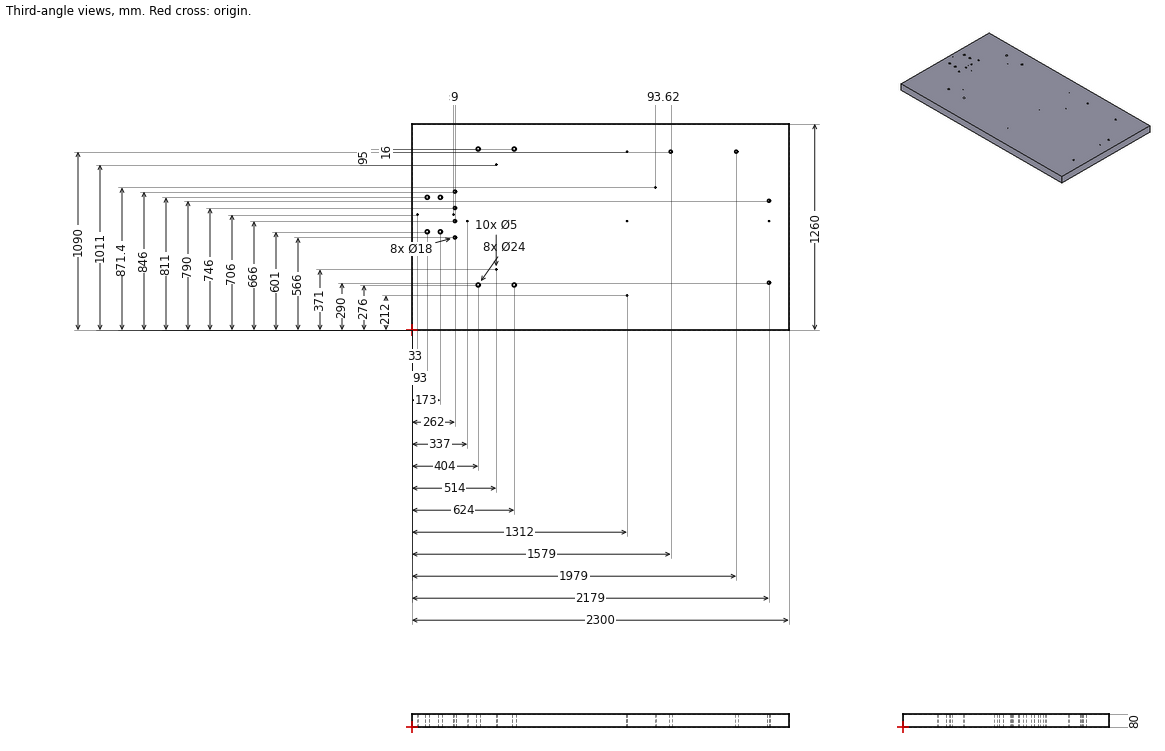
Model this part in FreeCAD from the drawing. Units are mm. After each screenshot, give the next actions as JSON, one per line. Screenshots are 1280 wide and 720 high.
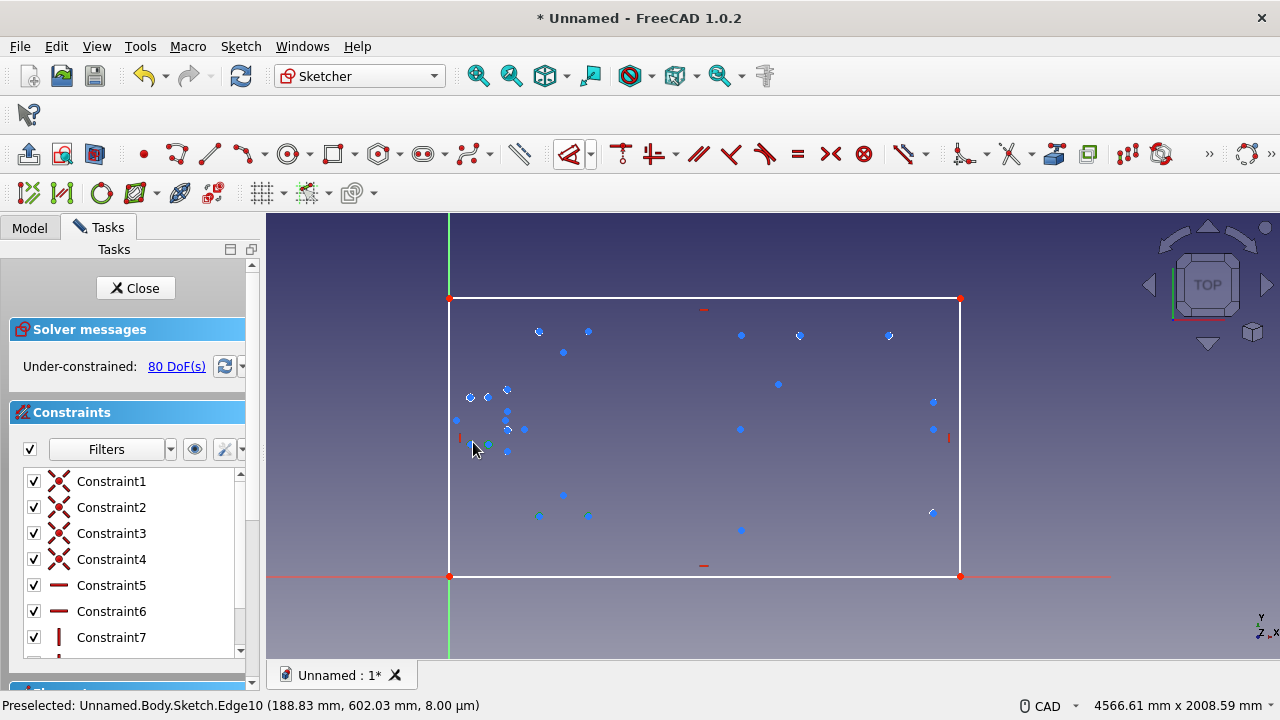
{"action": "scroll", "coordinate": [473, 395], "scroll_direction": "up", "scroll_amount": 8}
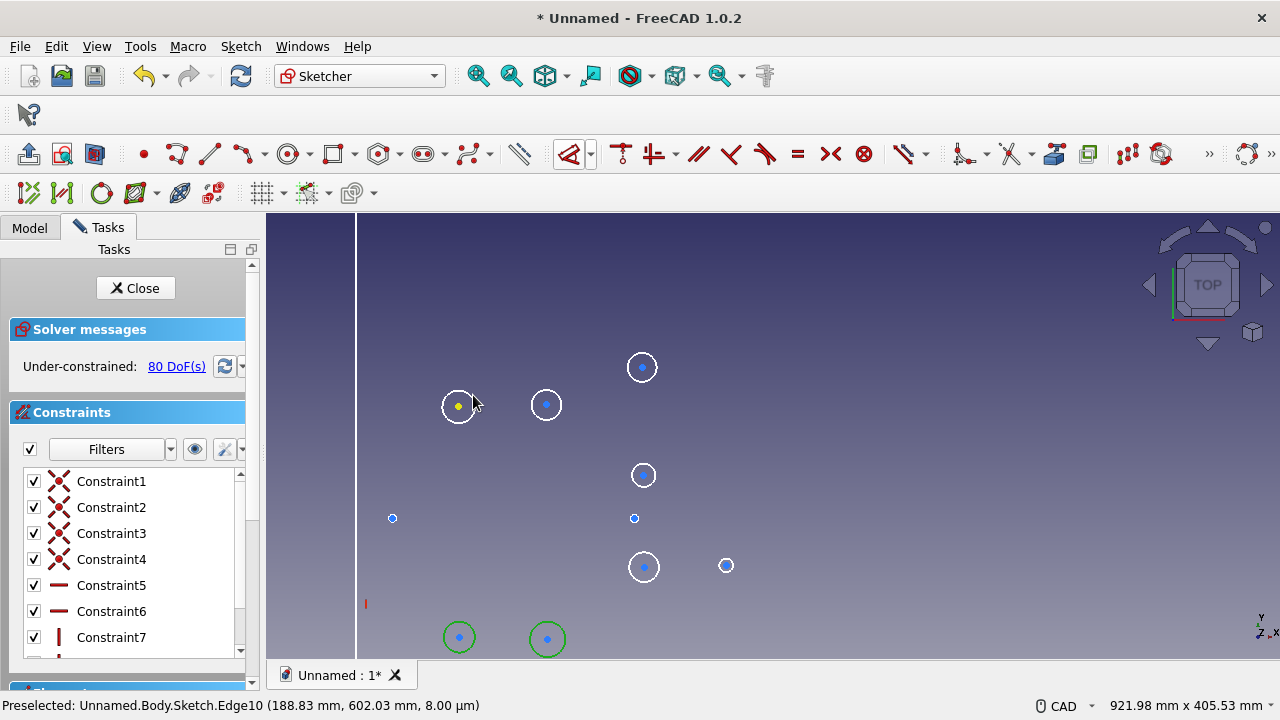
{"action": "left_click", "coordinate": [470, 395]}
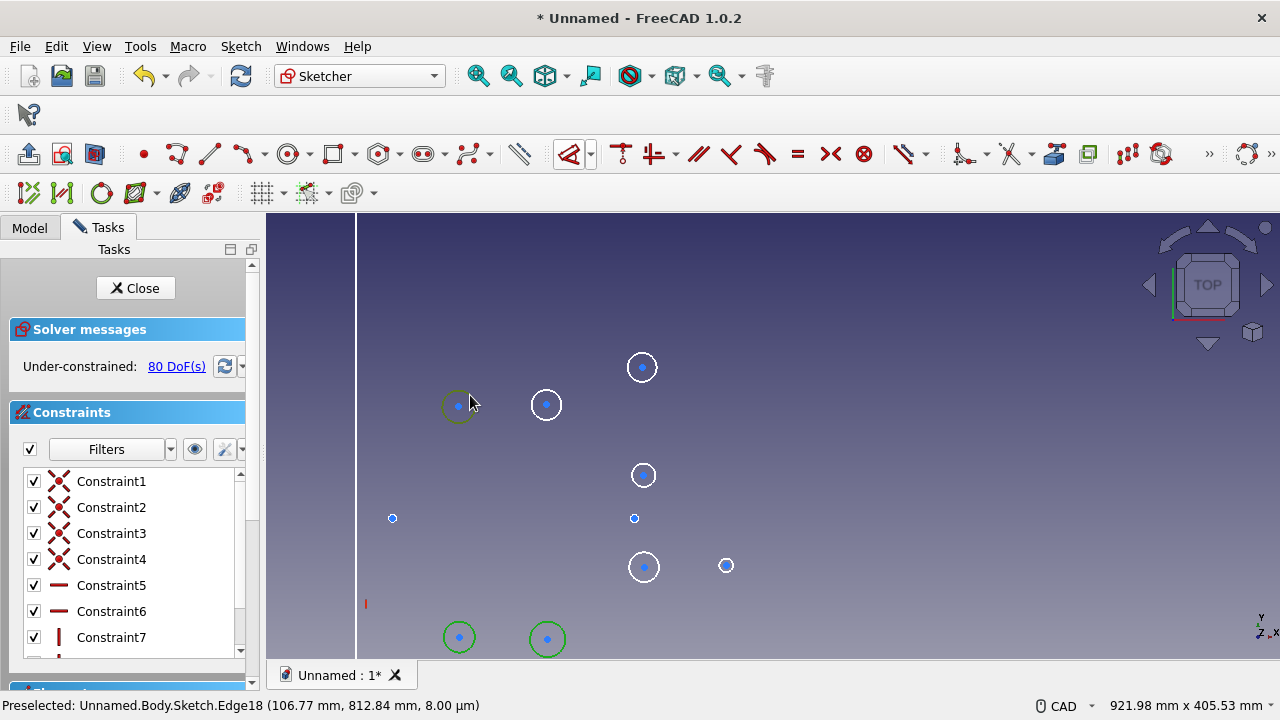
{"action": "left_click", "coordinate": [557, 394]}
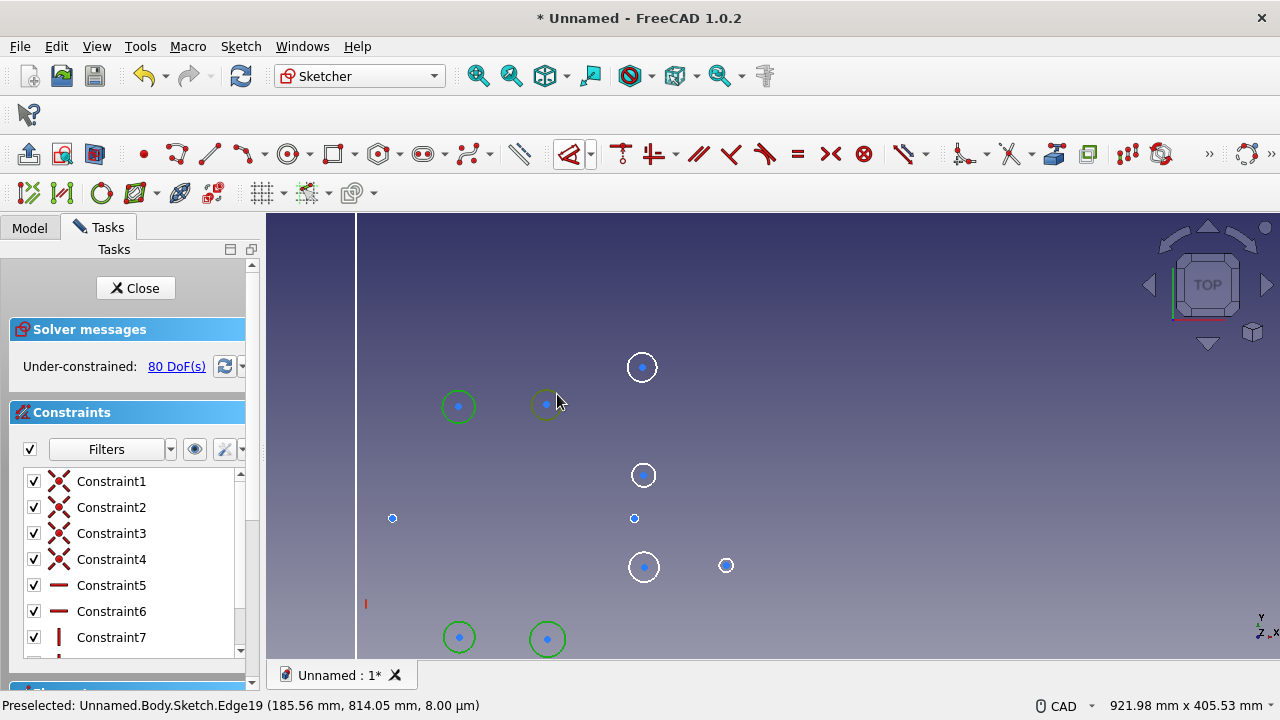
{"action": "scroll", "coordinate": [473, 394], "scroll_direction": "down", "scroll_amount": 8}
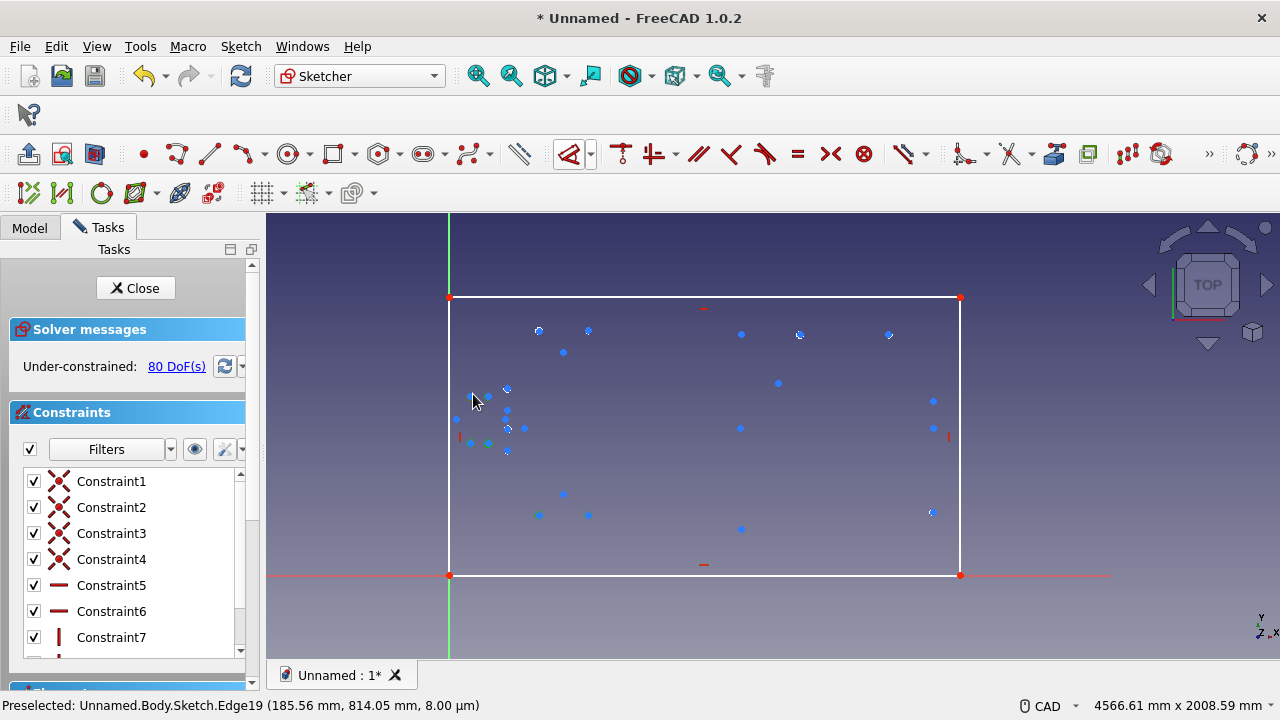
{"action": "scroll", "coordinate": [541, 329], "scroll_direction": "up", "scroll_amount": 8}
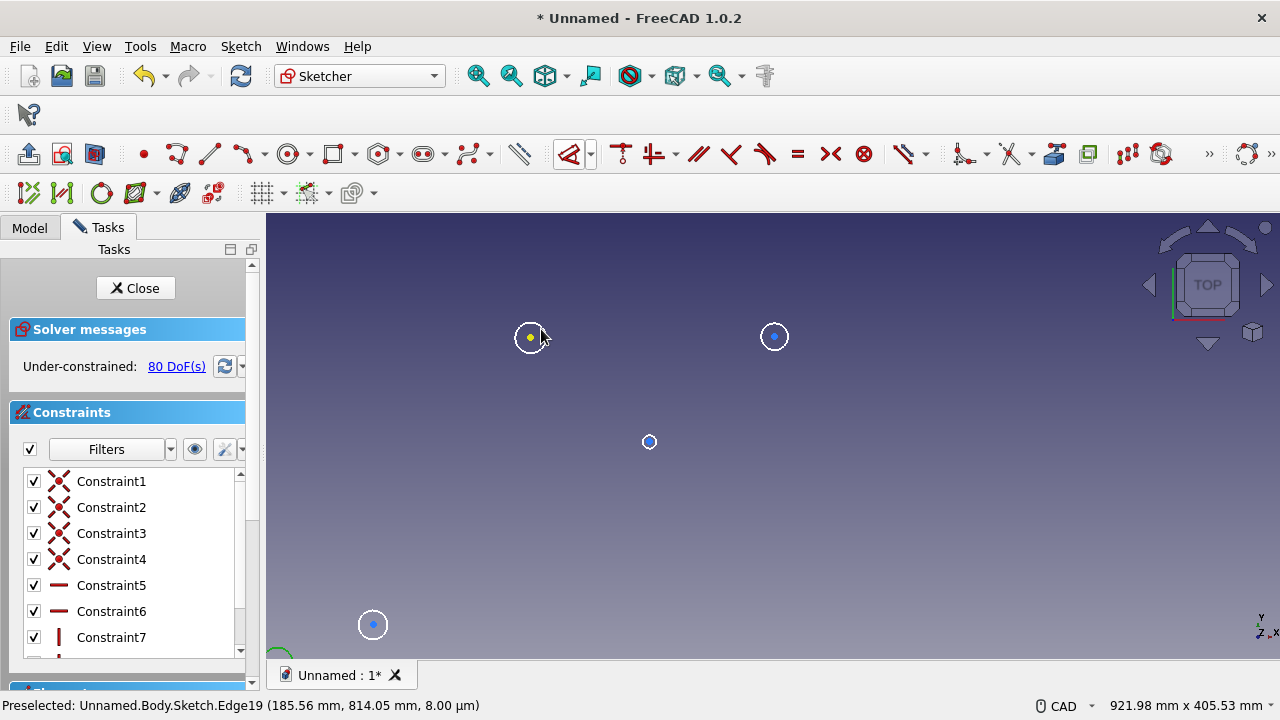
{"action": "left_click", "coordinate": [542, 327]}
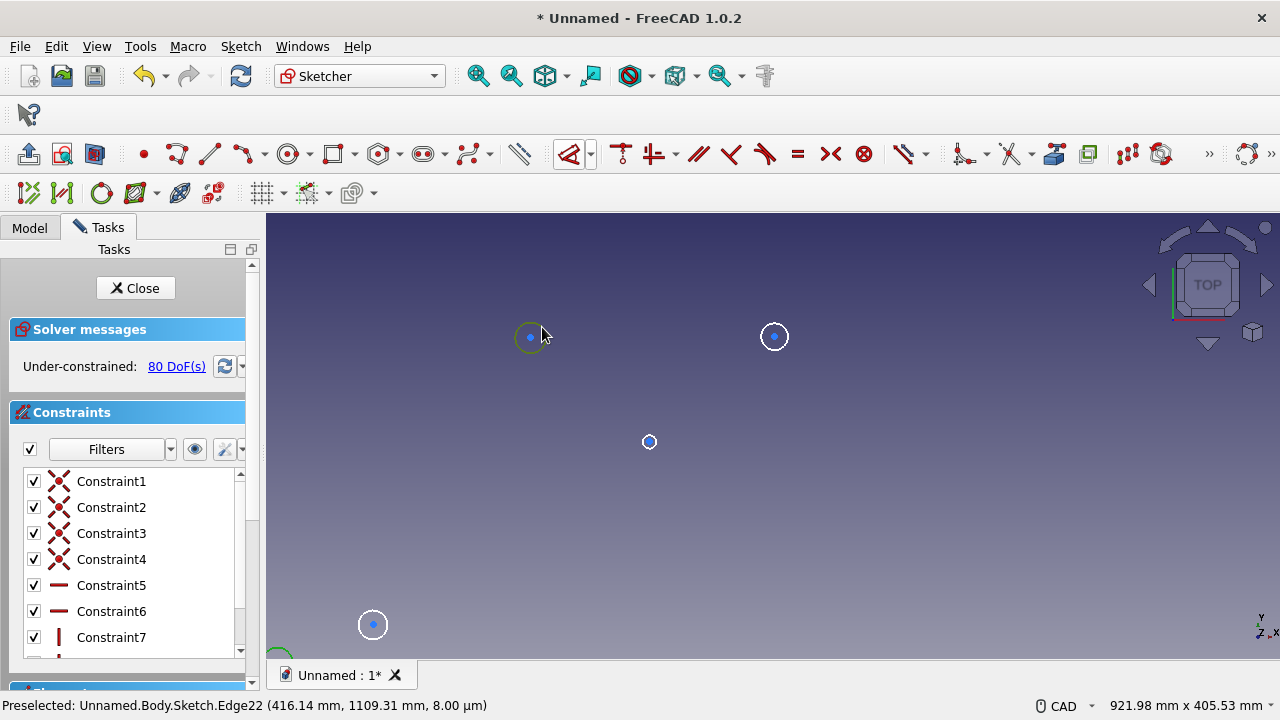
{"action": "left_click", "coordinate": [784, 327]}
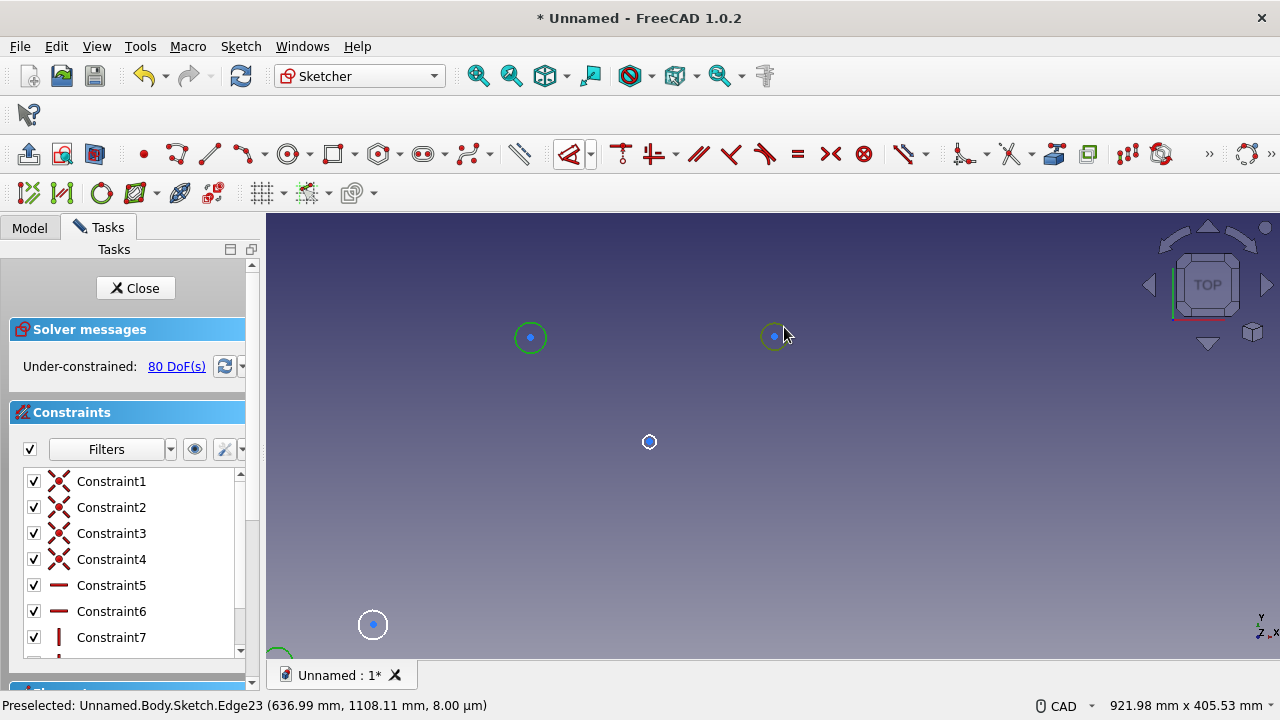
{"action": "left_click", "coordinate": [798, 154]}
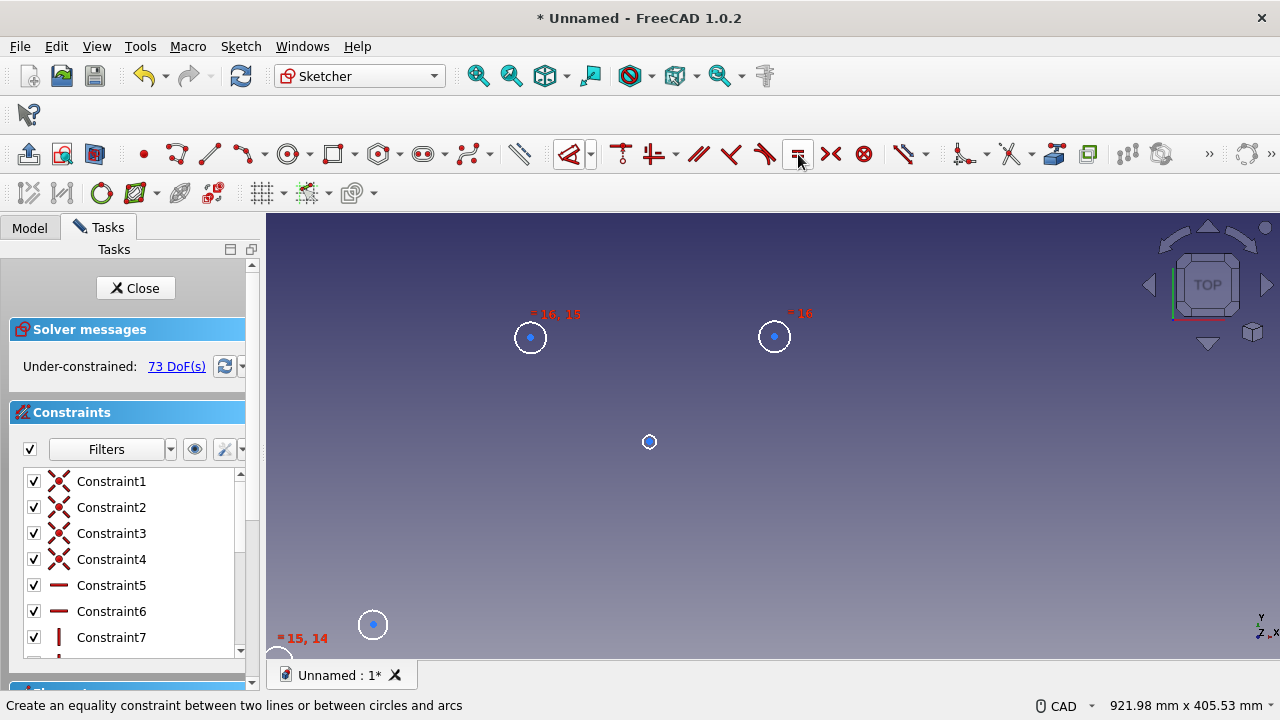
{"action": "scroll", "coordinate": [541, 329], "scroll_direction": "down", "scroll_amount": 8}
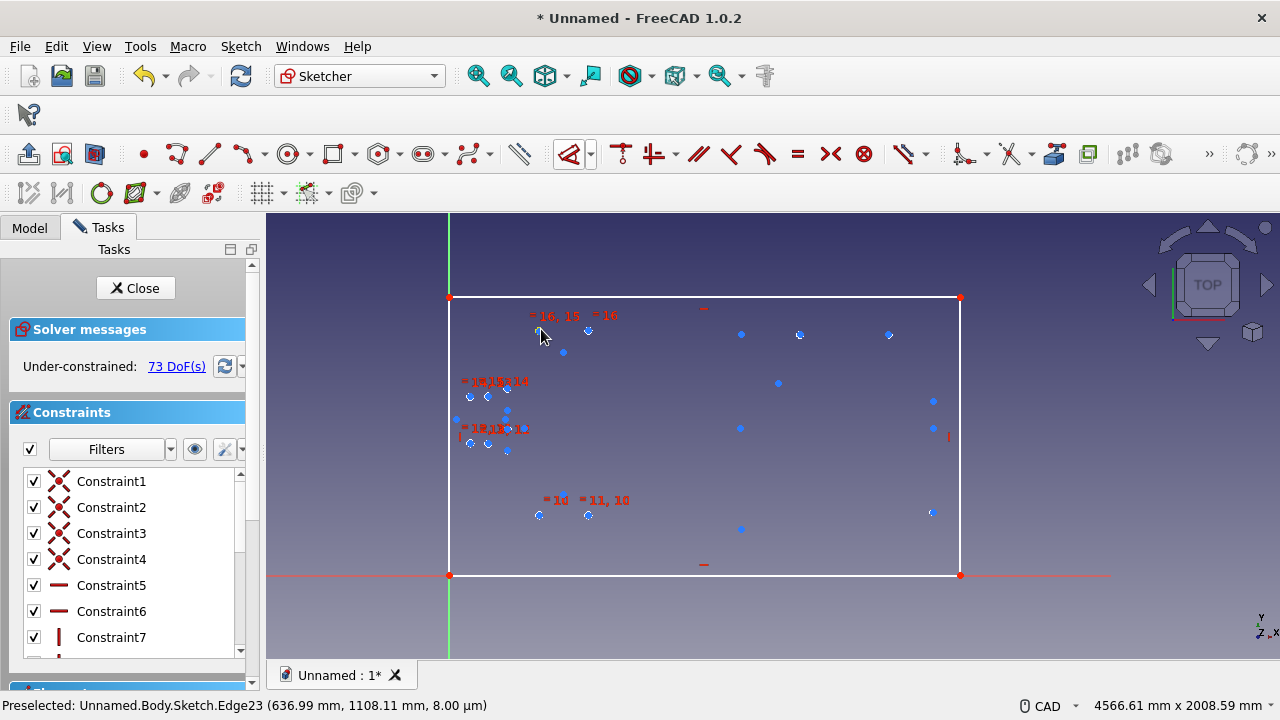
{"action": "scroll", "coordinate": [565, 494], "scroll_direction": "up", "scroll_amount": 12}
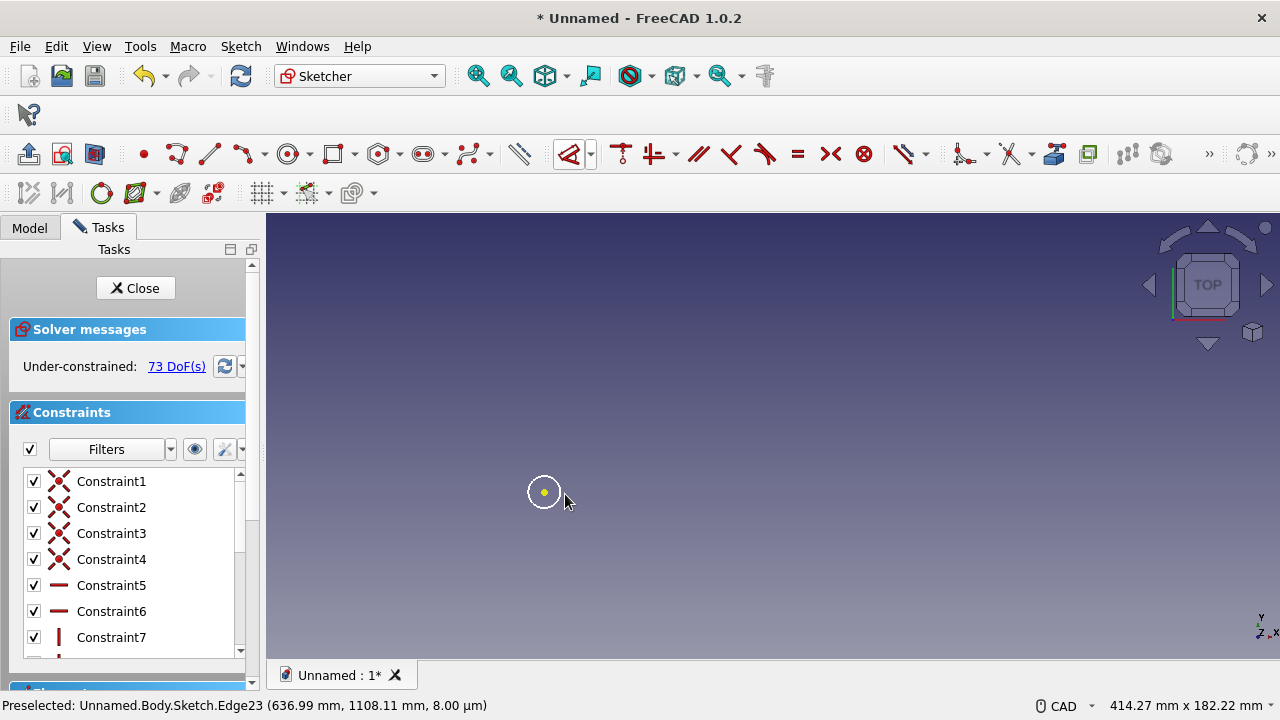
{"action": "left_click", "coordinate": [560, 493]}